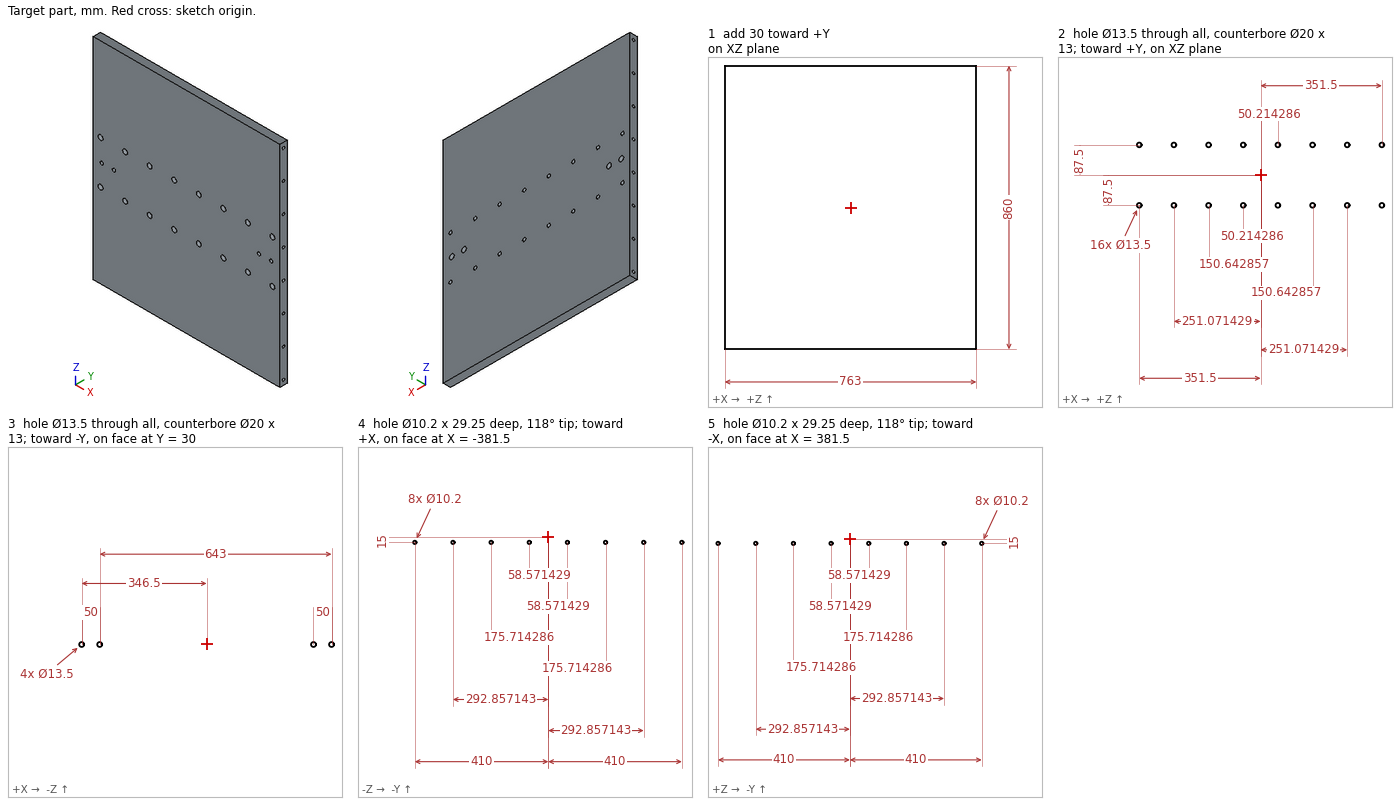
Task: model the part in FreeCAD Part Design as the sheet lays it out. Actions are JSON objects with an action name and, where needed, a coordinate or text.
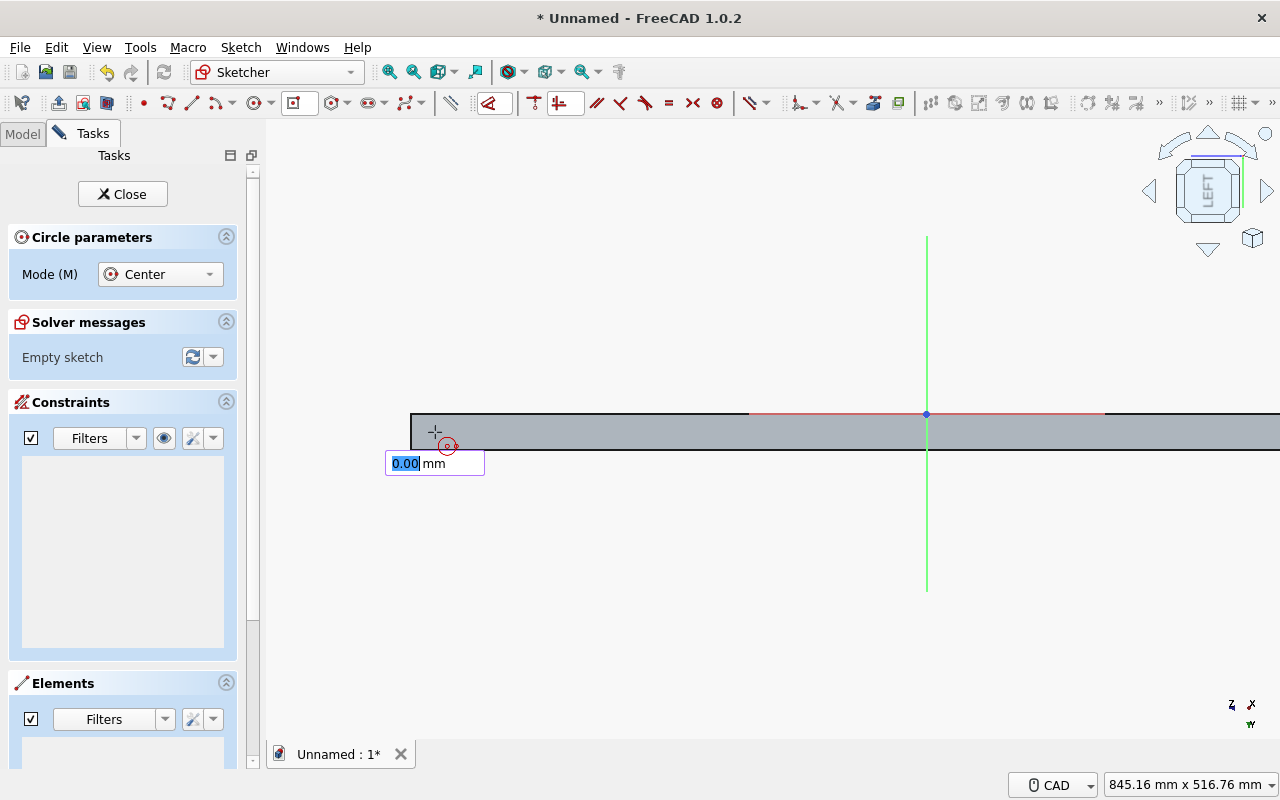
{"action": "scroll", "coordinate": [439, 437], "scroll_direction": "up", "scroll_amount": 5}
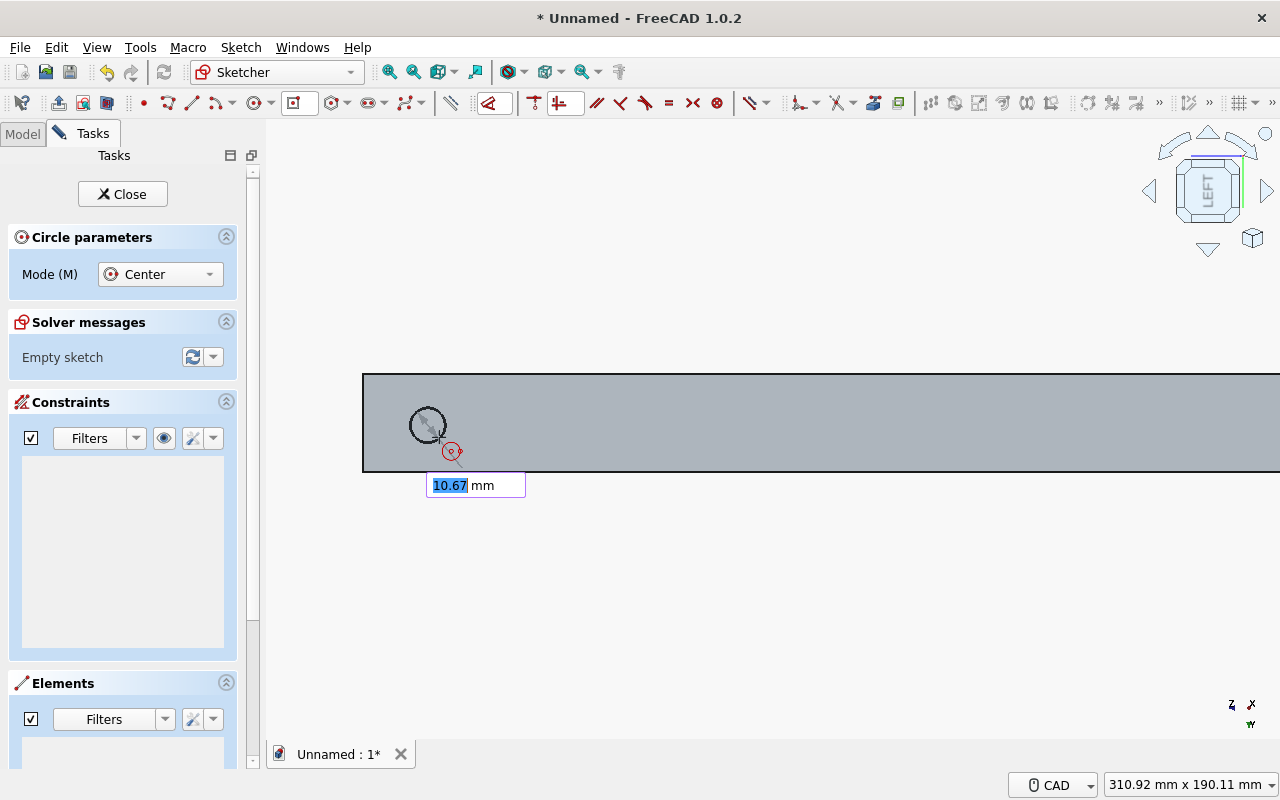
{"action": "left_click", "coordinate": [440, 435]}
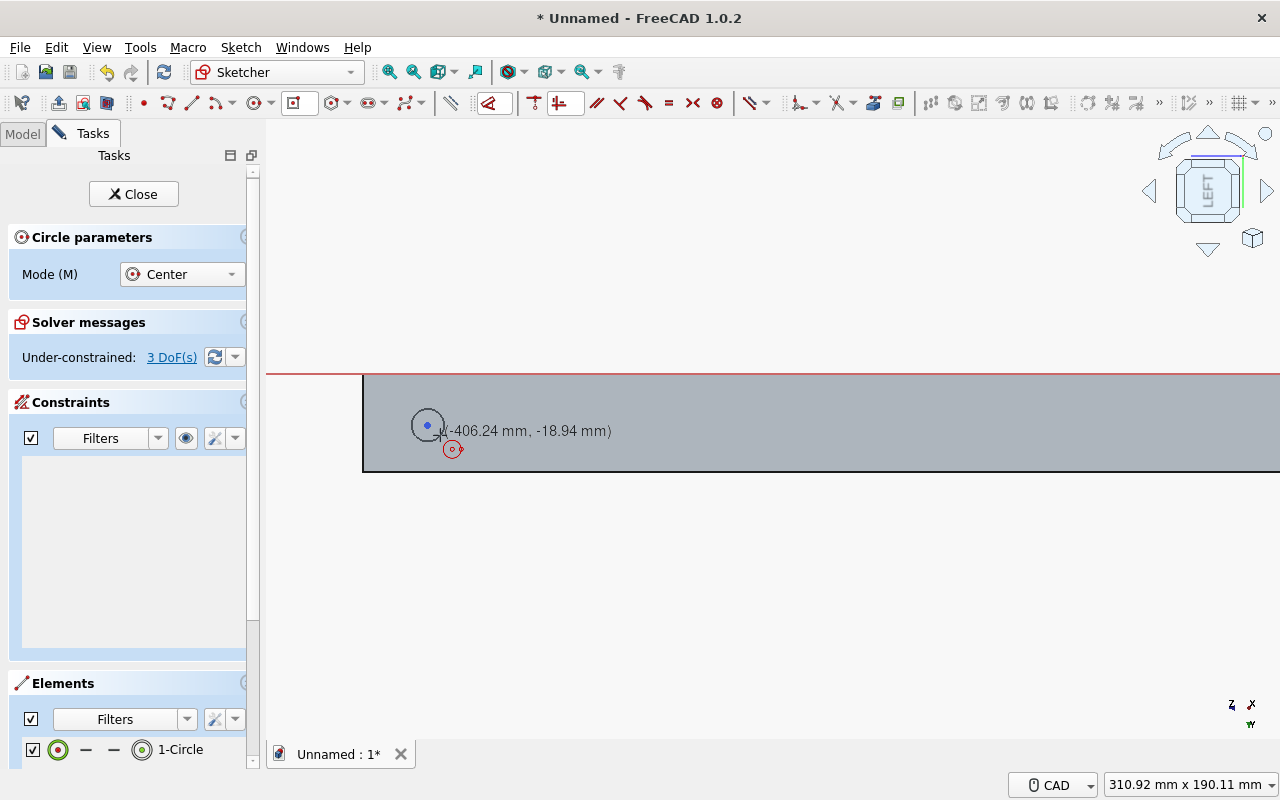
{"action": "scroll", "coordinate": [810, 423], "scroll_direction": "up", "scroll_amount": 2}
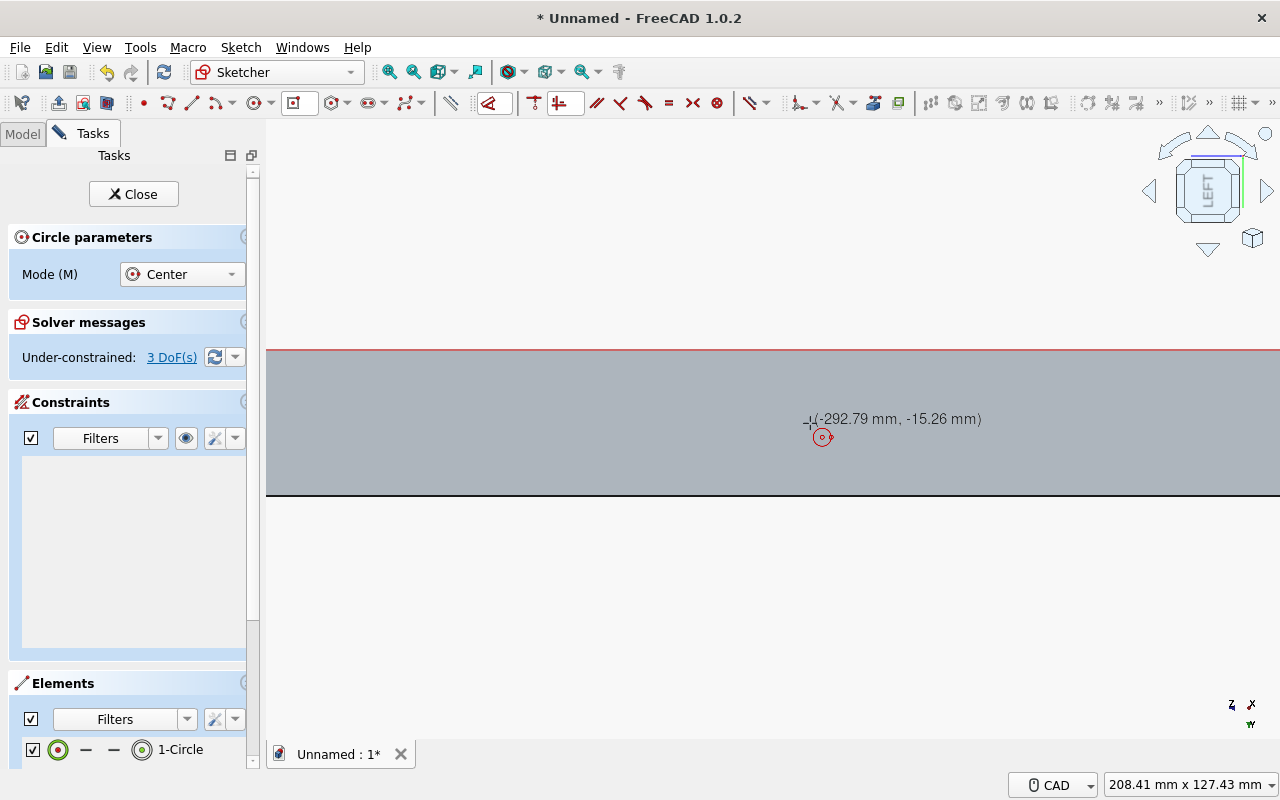
{"action": "scroll", "coordinate": [465, 434], "scroll_direction": "down", "scroll_amount": 10}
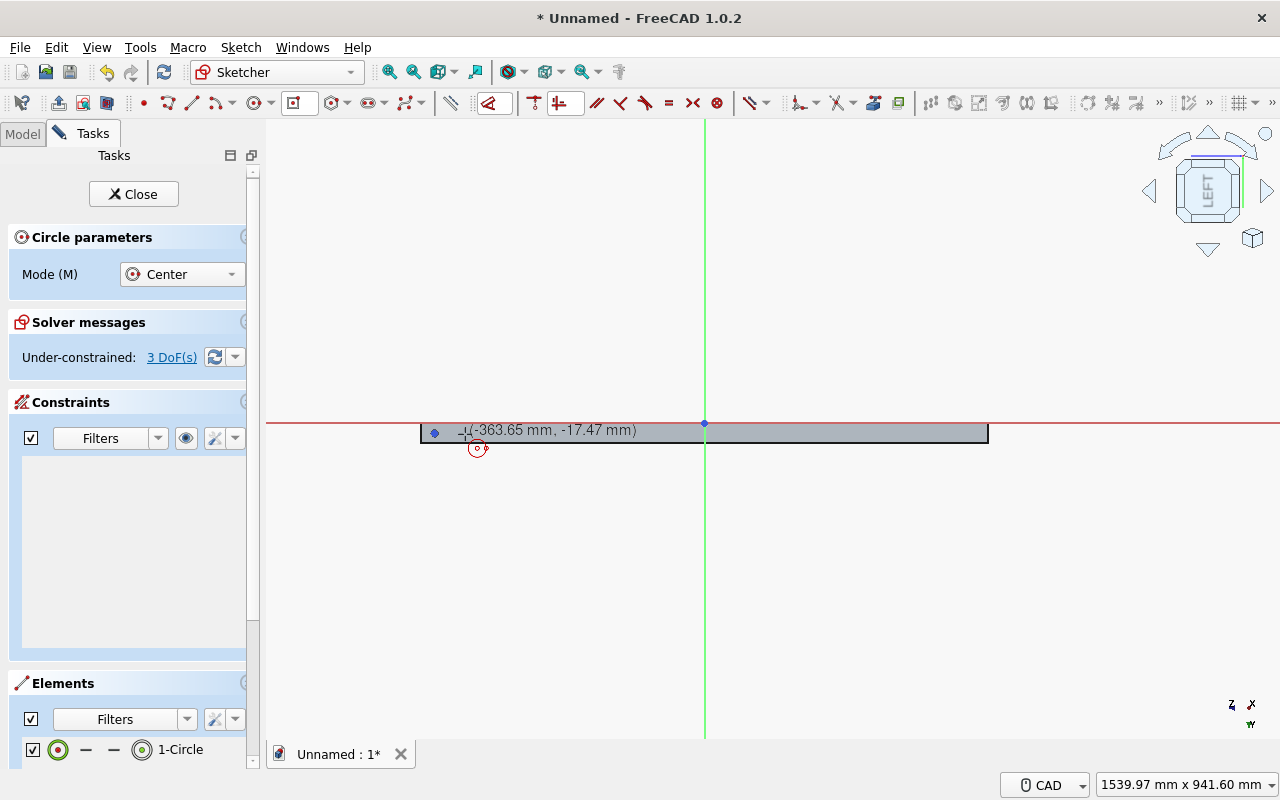
{"action": "scroll", "coordinate": [512, 433], "scroll_direction": "up", "scroll_amount": 3}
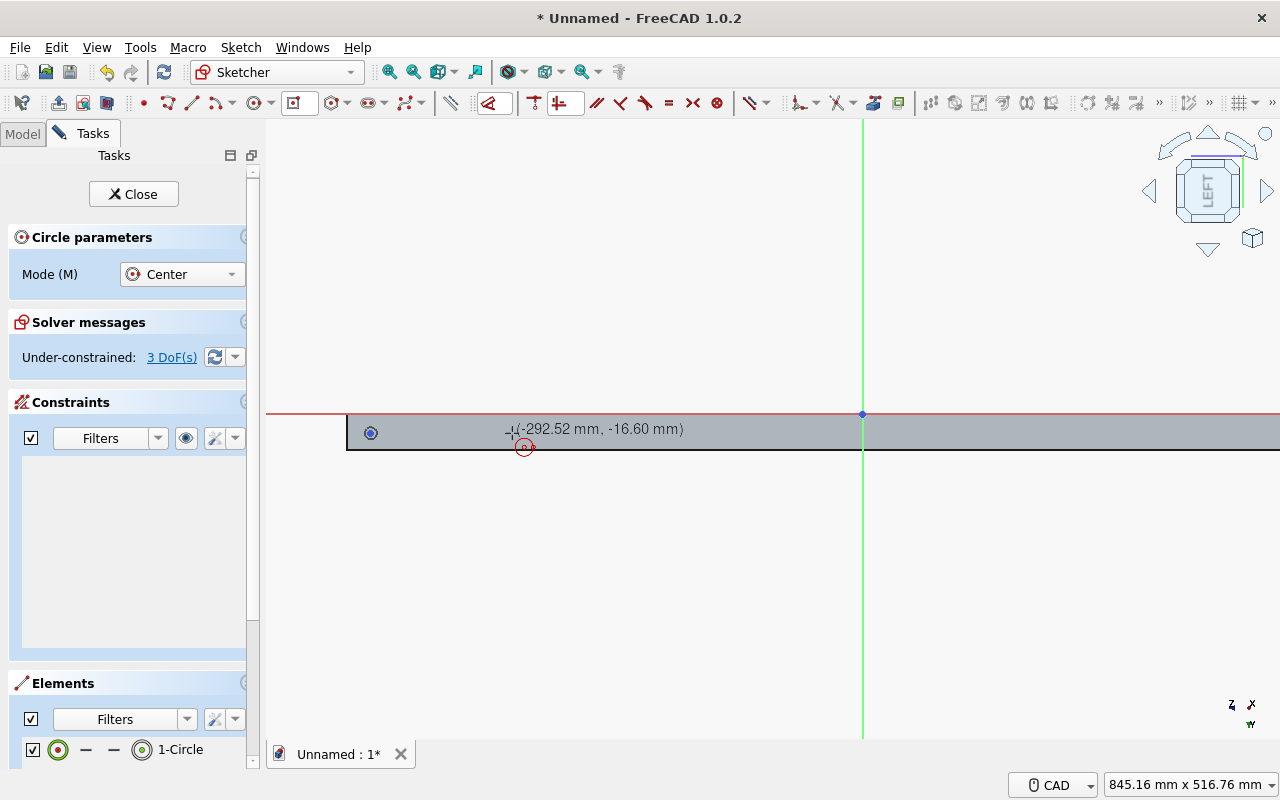
{"action": "left_click", "coordinate": [511, 432]}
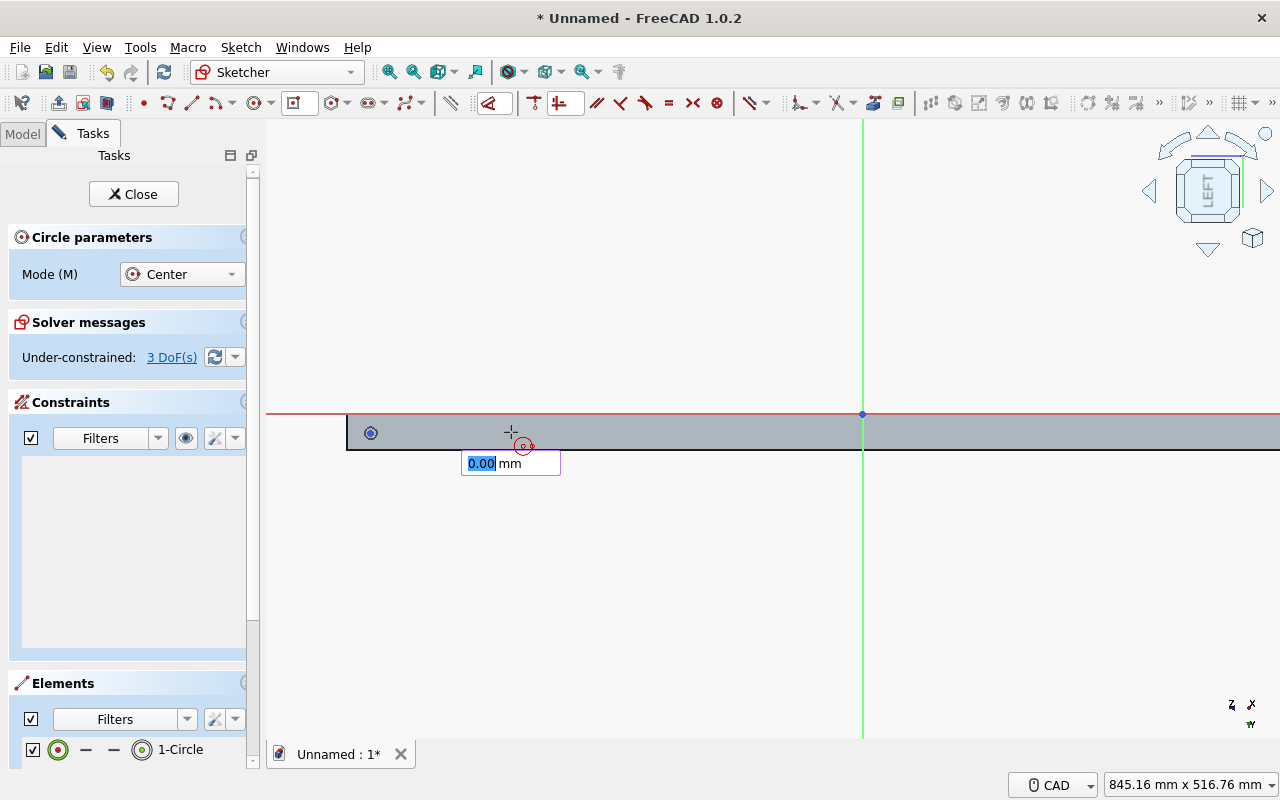
{"action": "scroll", "coordinate": [516, 437], "scroll_direction": "up", "scroll_amount": 5}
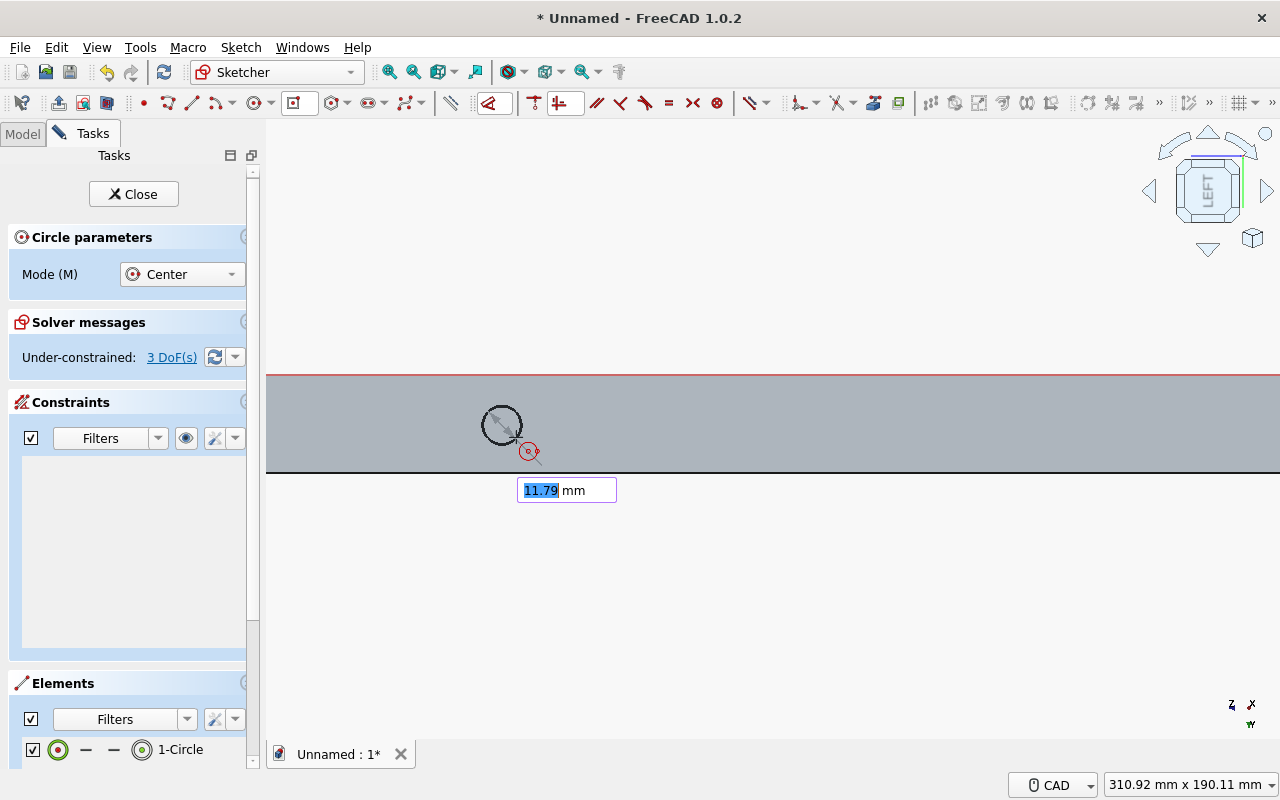
{"action": "left_click", "coordinate": [515, 436]}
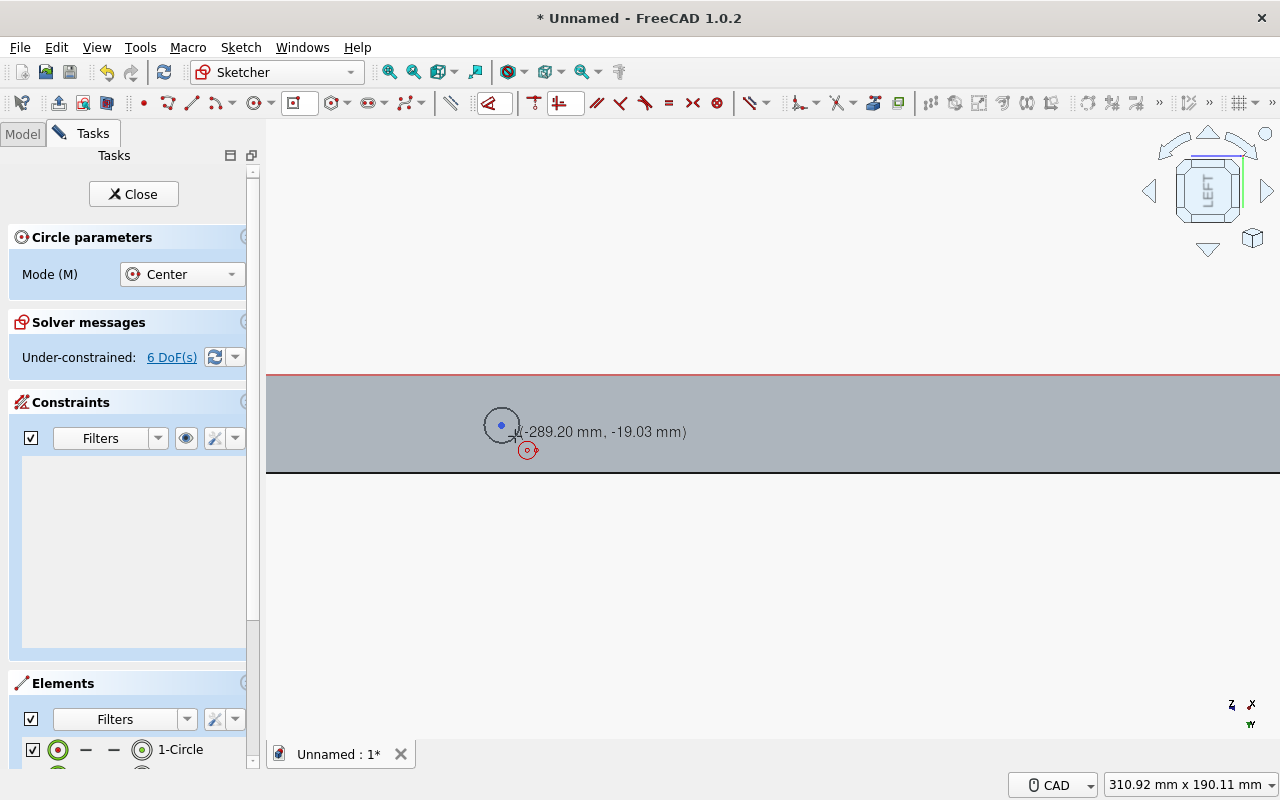
{"action": "scroll", "coordinate": [885, 424], "scroll_direction": "up", "scroll_amount": 2}